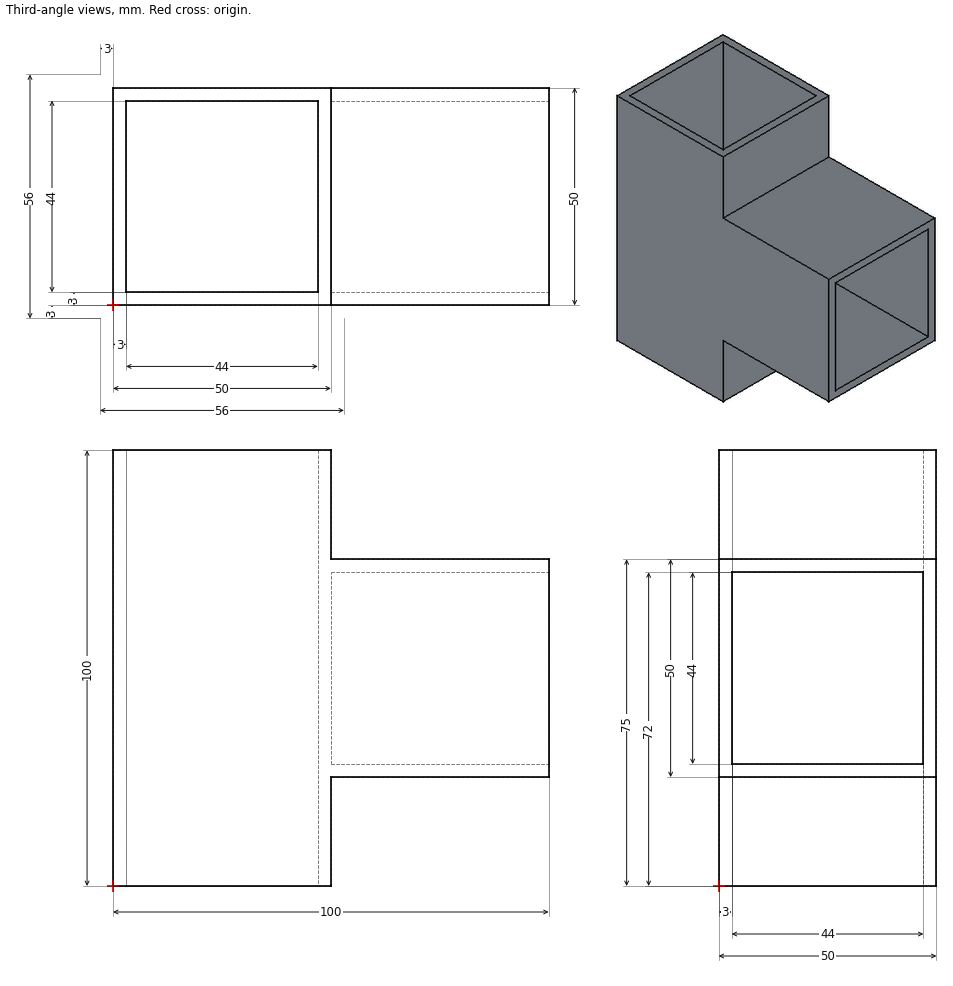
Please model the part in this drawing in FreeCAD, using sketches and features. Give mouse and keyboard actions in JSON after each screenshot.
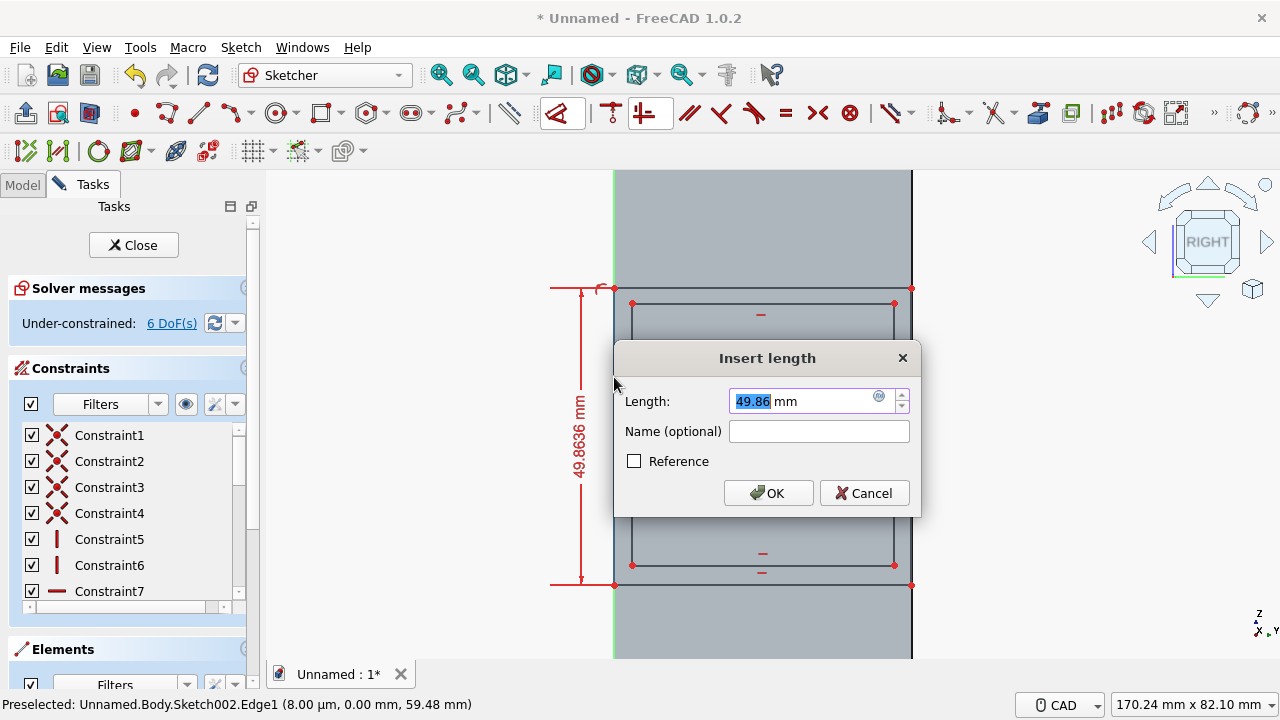
{"action": "type", "text": "50"}
{"action": "key", "text": "Return"}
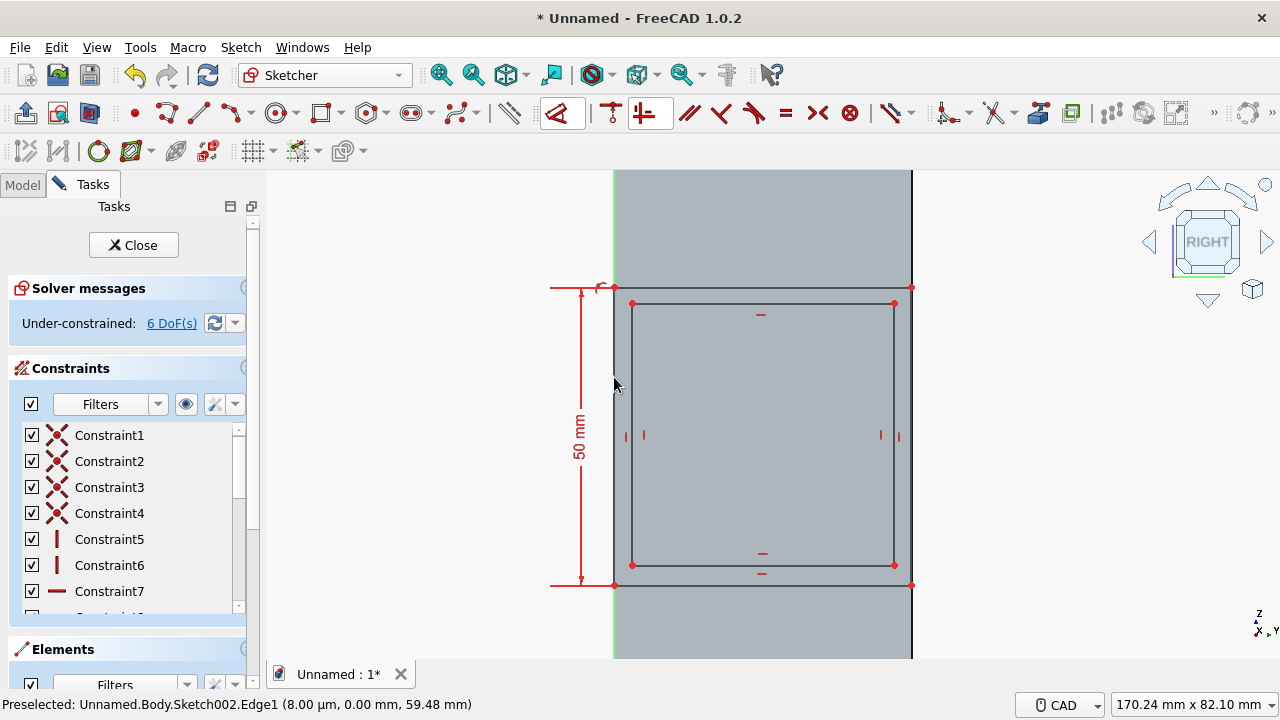
{"action": "left_click", "coordinate": [703, 586]}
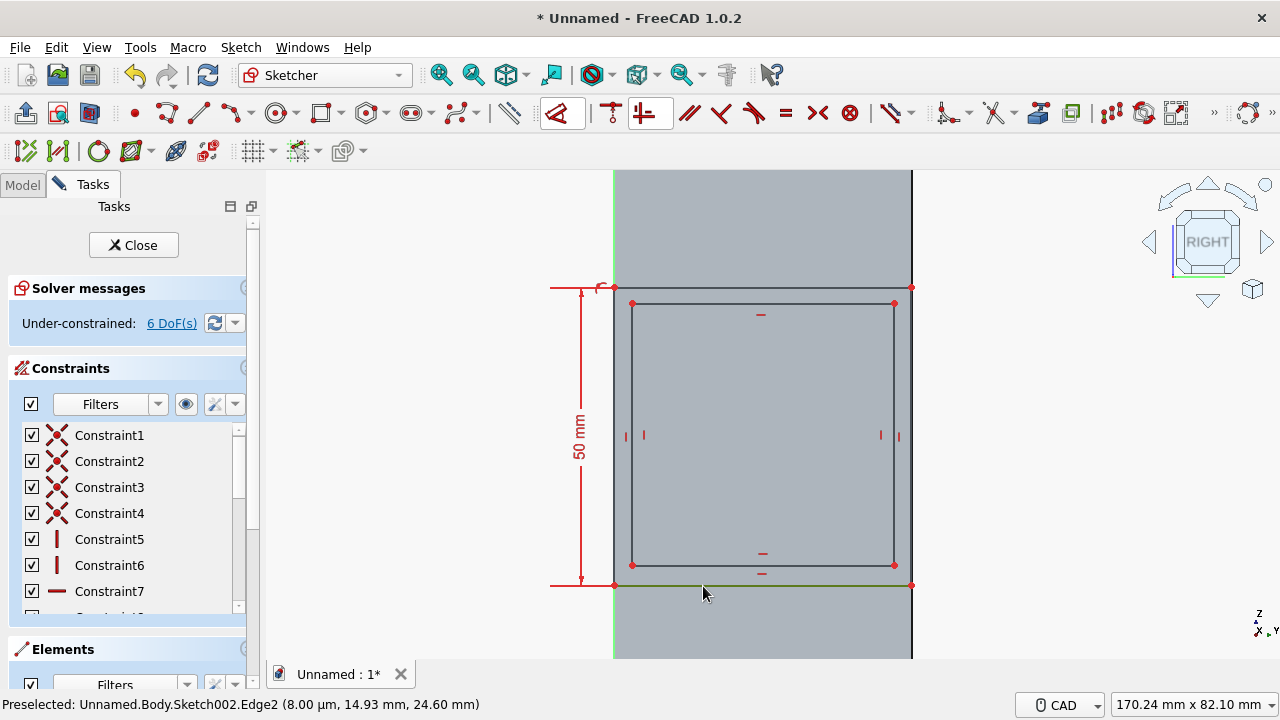
{"action": "key", "text": "l"}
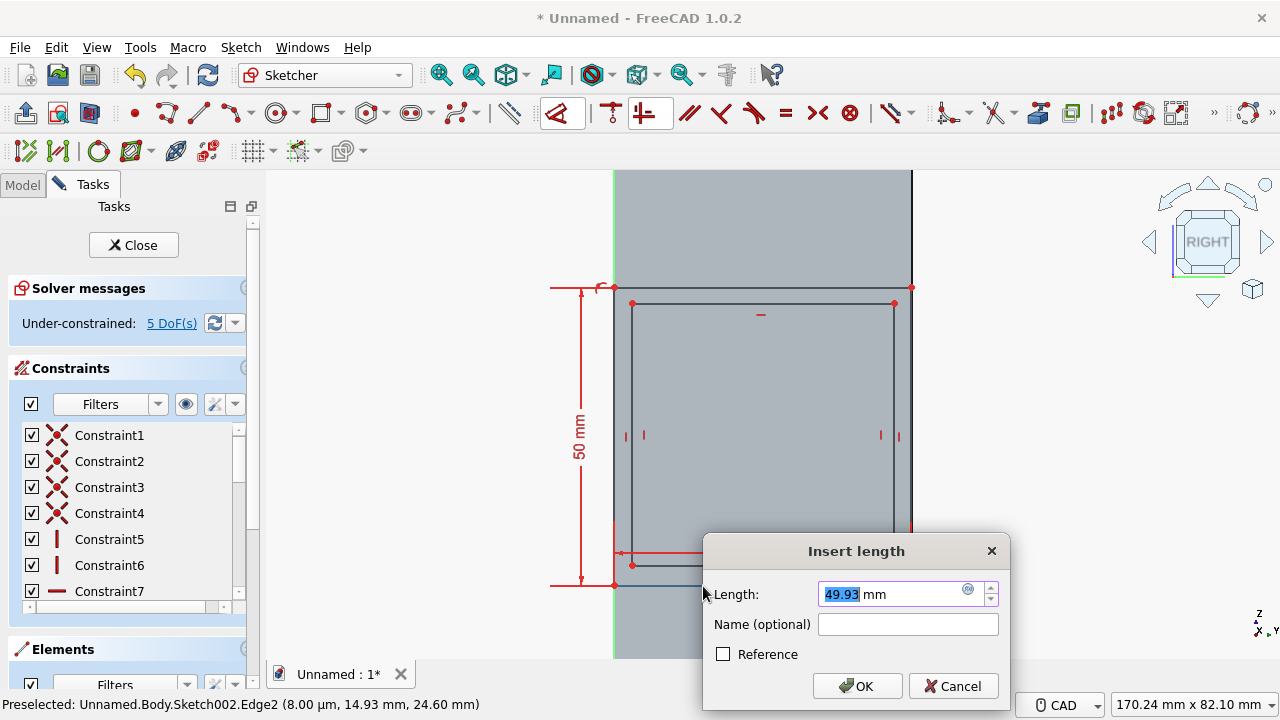
{"action": "type", "text": "50"}
{"action": "key", "text": "Return"}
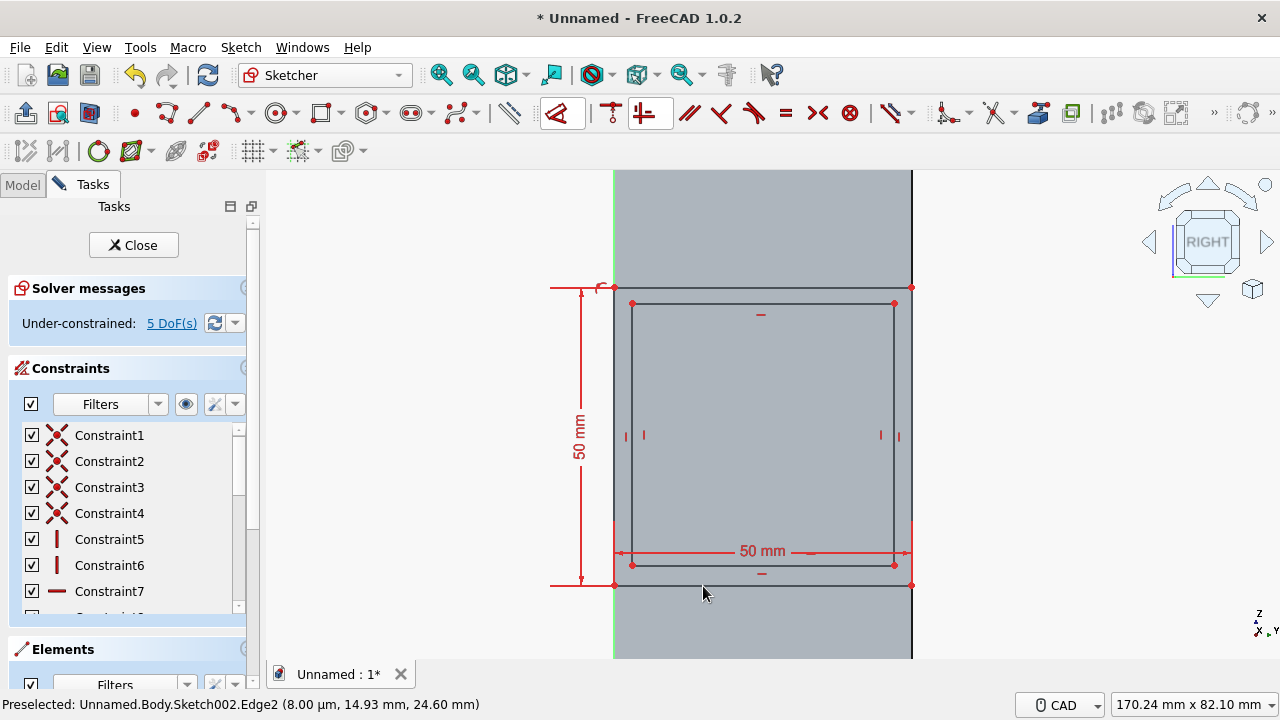
{"action": "left_click", "coordinate": [632, 383]}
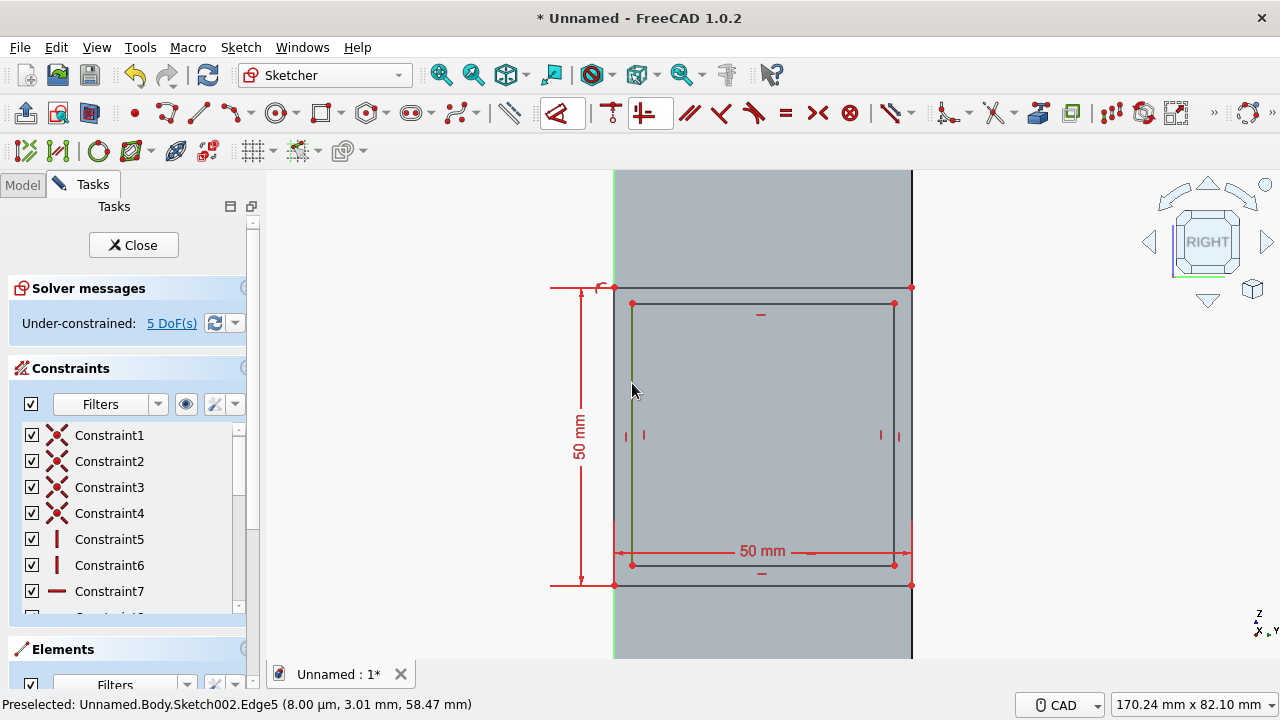
{"action": "key", "text": "i"}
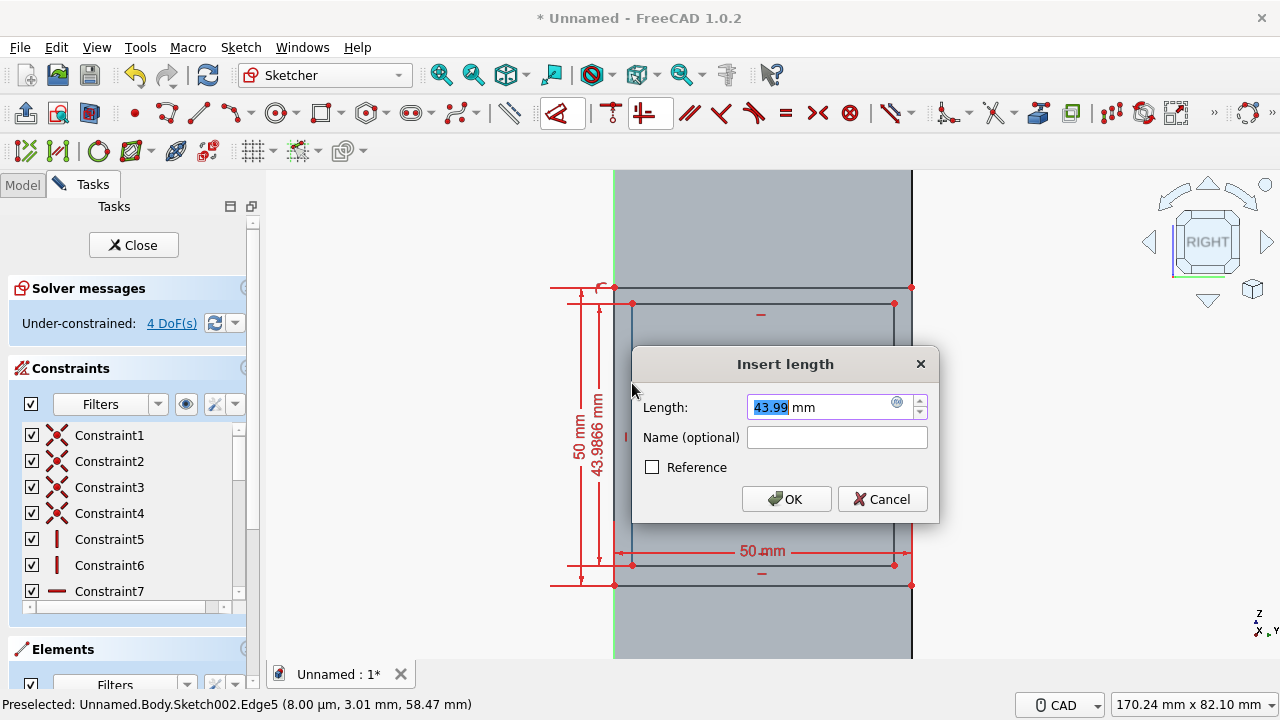
{"action": "type", "text": "44"}
{"action": "key", "text": "Return"}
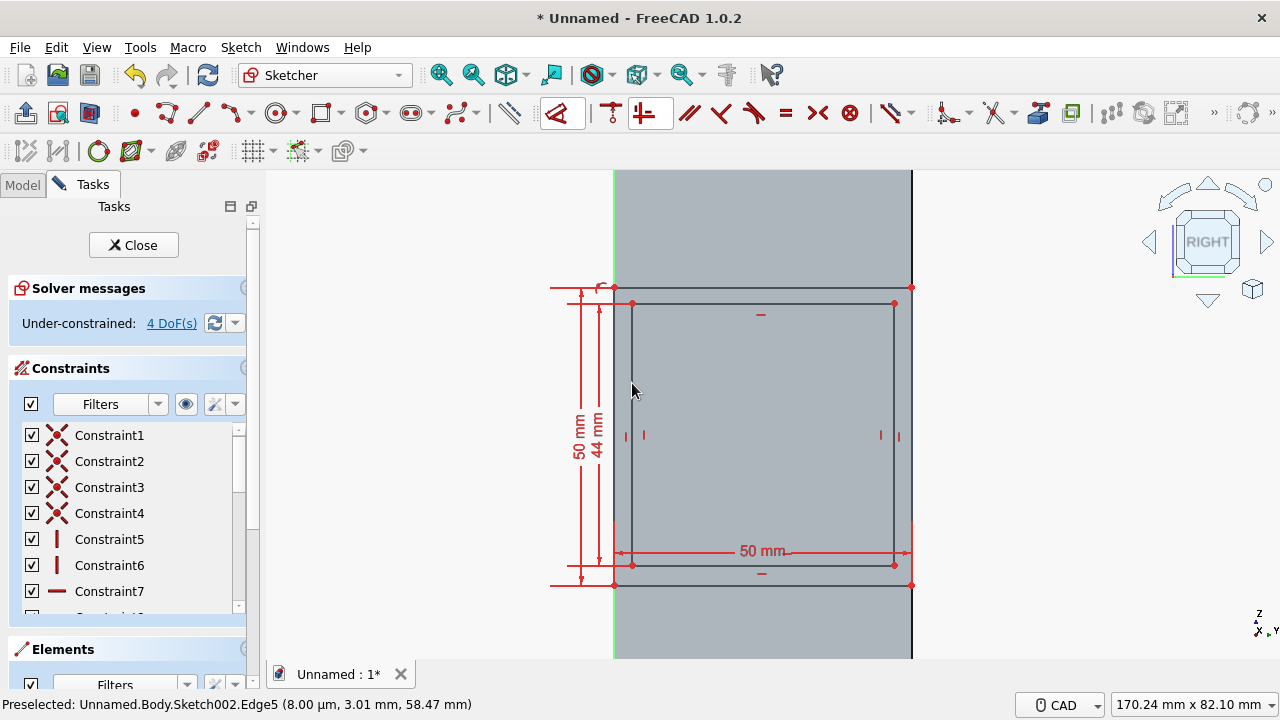
{"action": "left_click", "coordinate": [711, 566]}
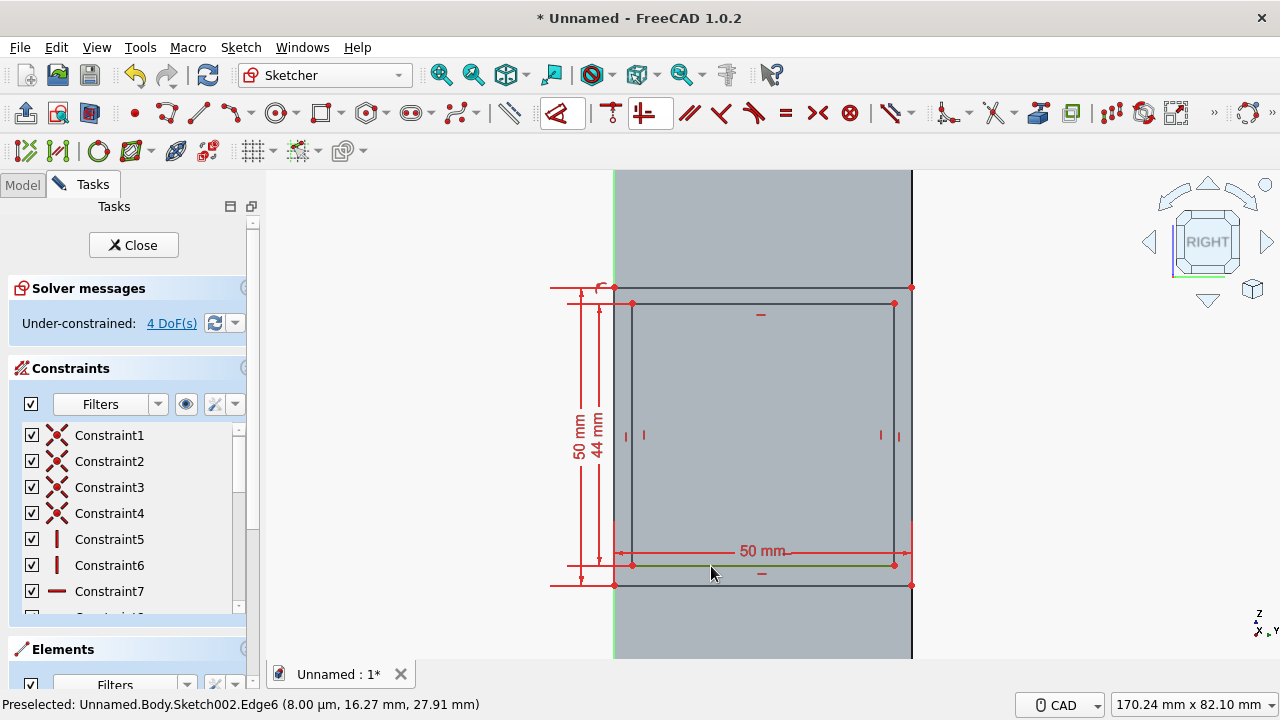
{"action": "key", "text": "l"}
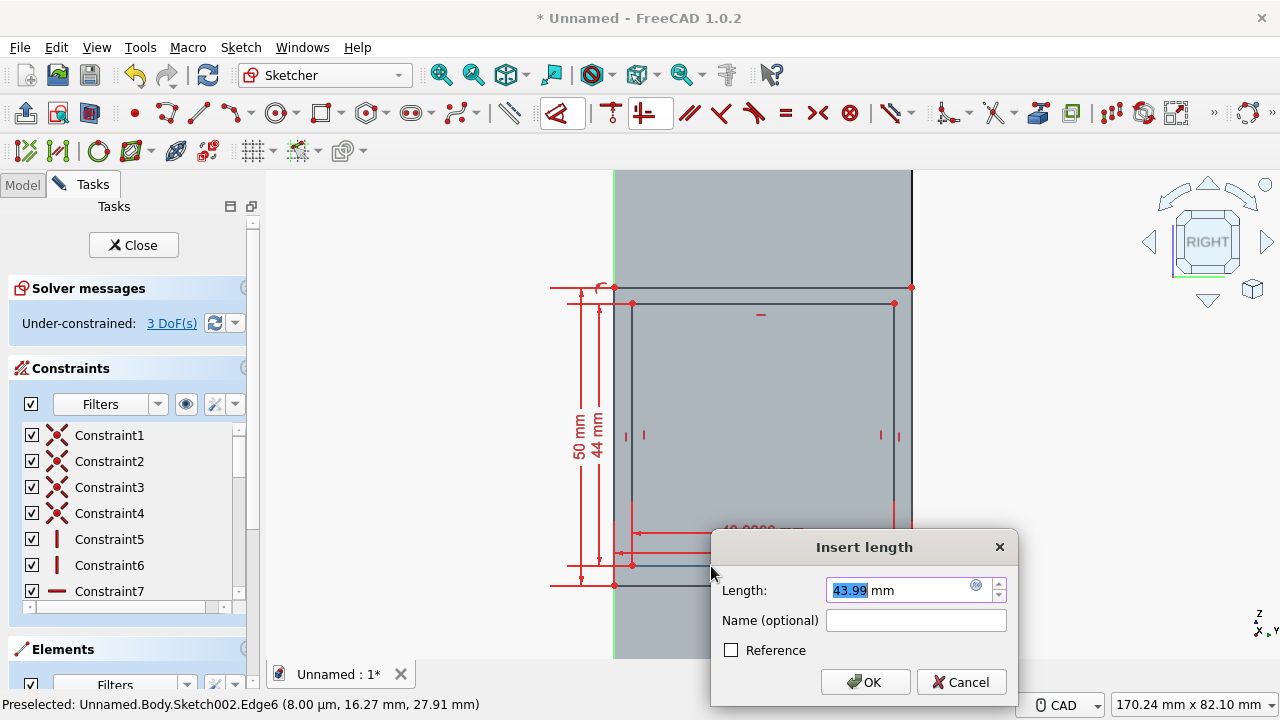
{"action": "type", "text": "44"}
{"action": "key", "text": "Return"}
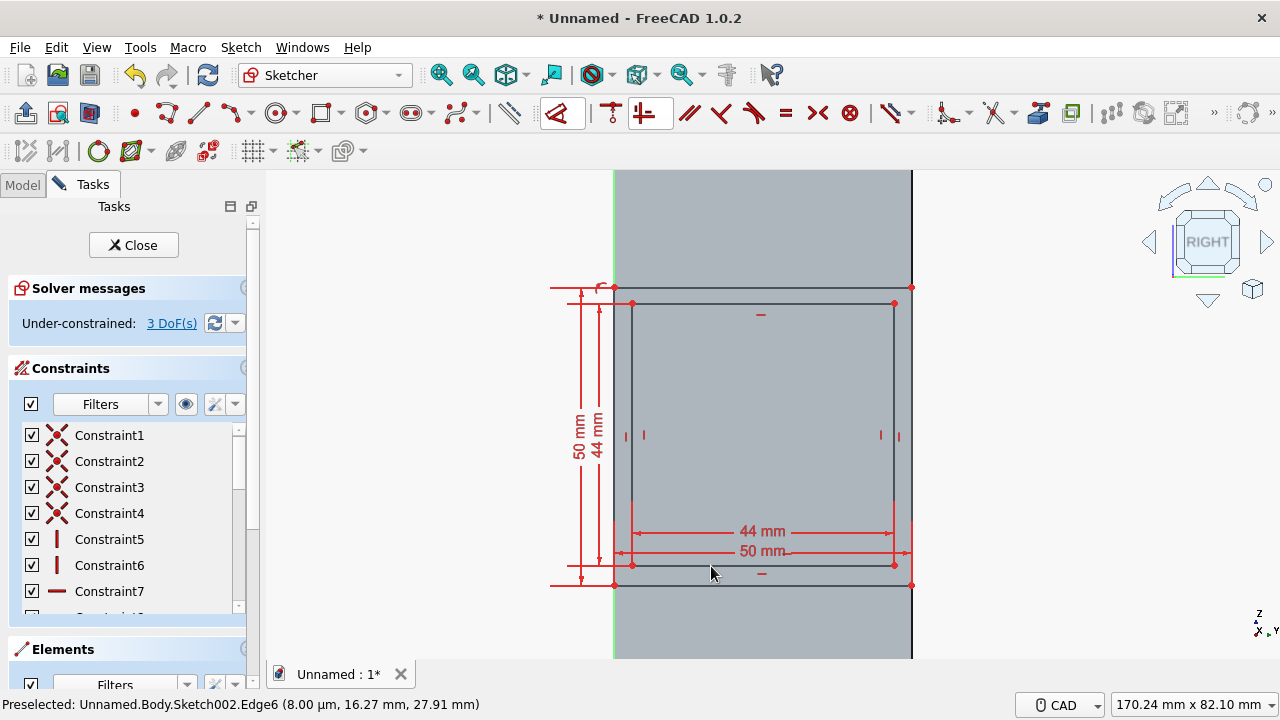
{"action": "scroll", "coordinate": [632, 304], "scroll_direction": "up", "scroll_amount": 4}